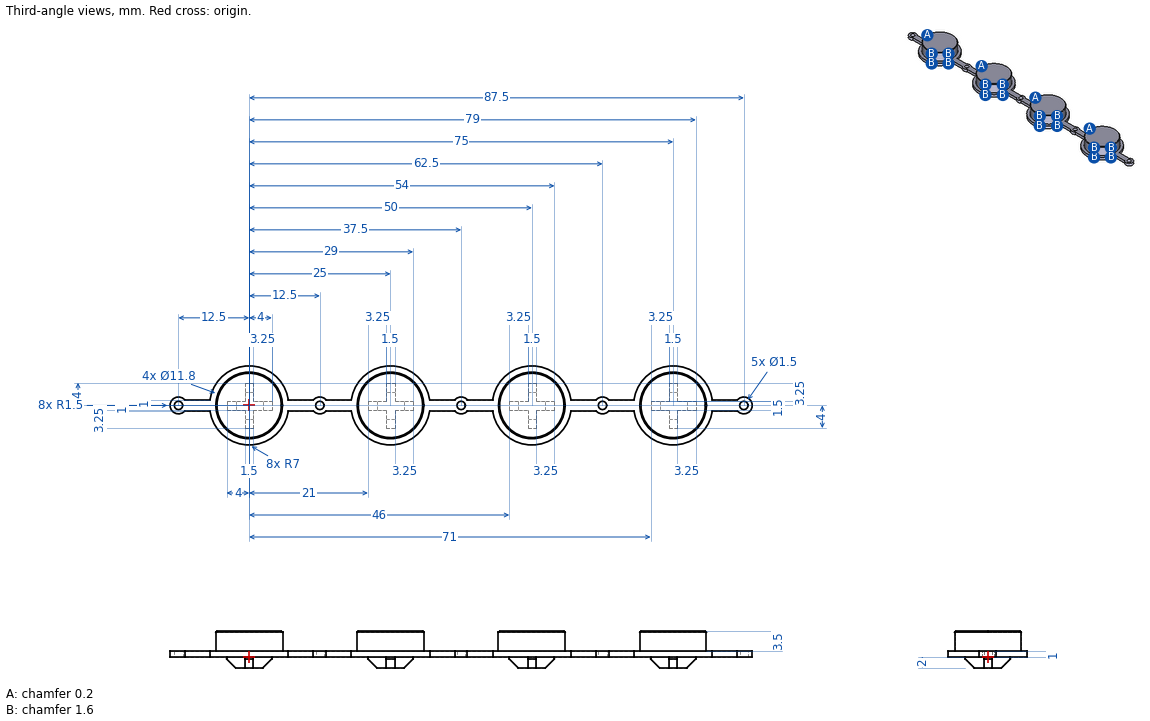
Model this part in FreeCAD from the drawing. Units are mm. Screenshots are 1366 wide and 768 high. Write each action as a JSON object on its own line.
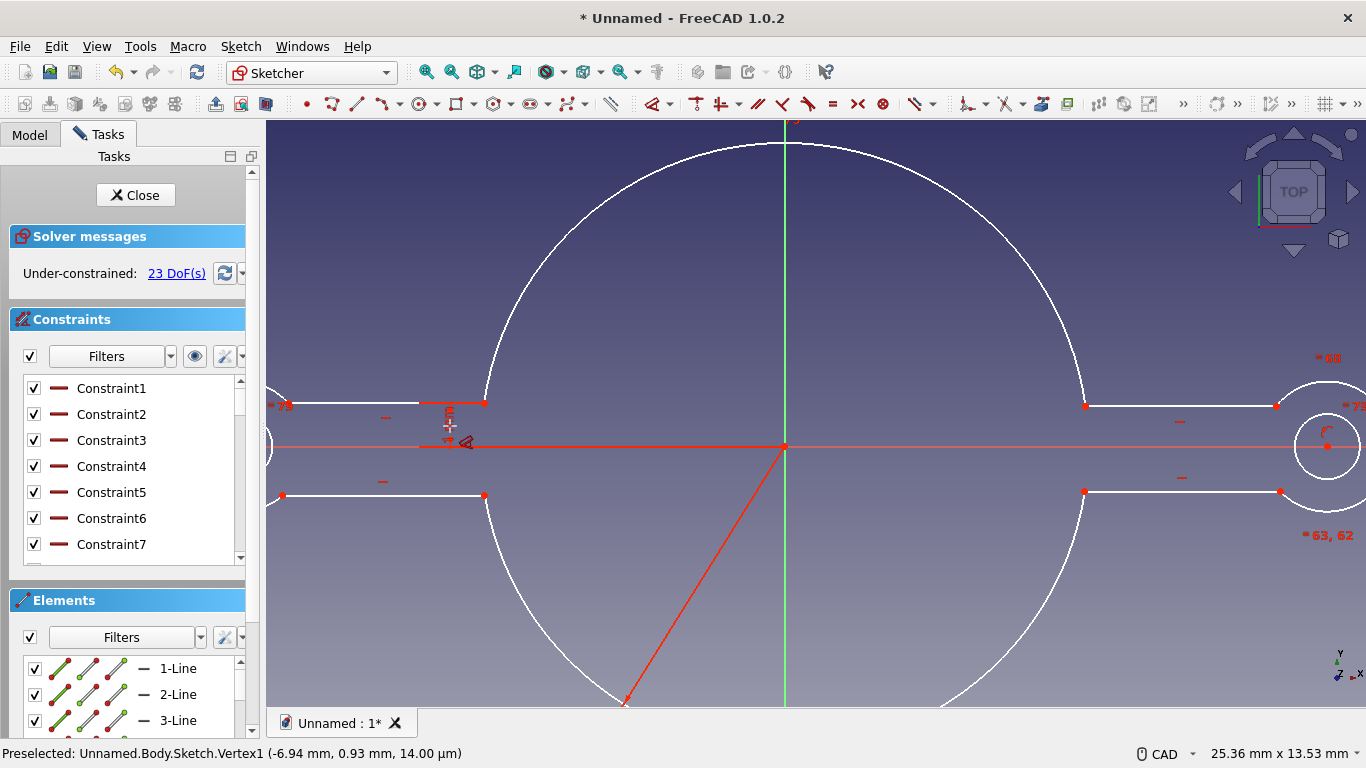
{"action": "scroll", "coordinate": [487, 408], "scroll_direction": "down", "scroll_amount": 10}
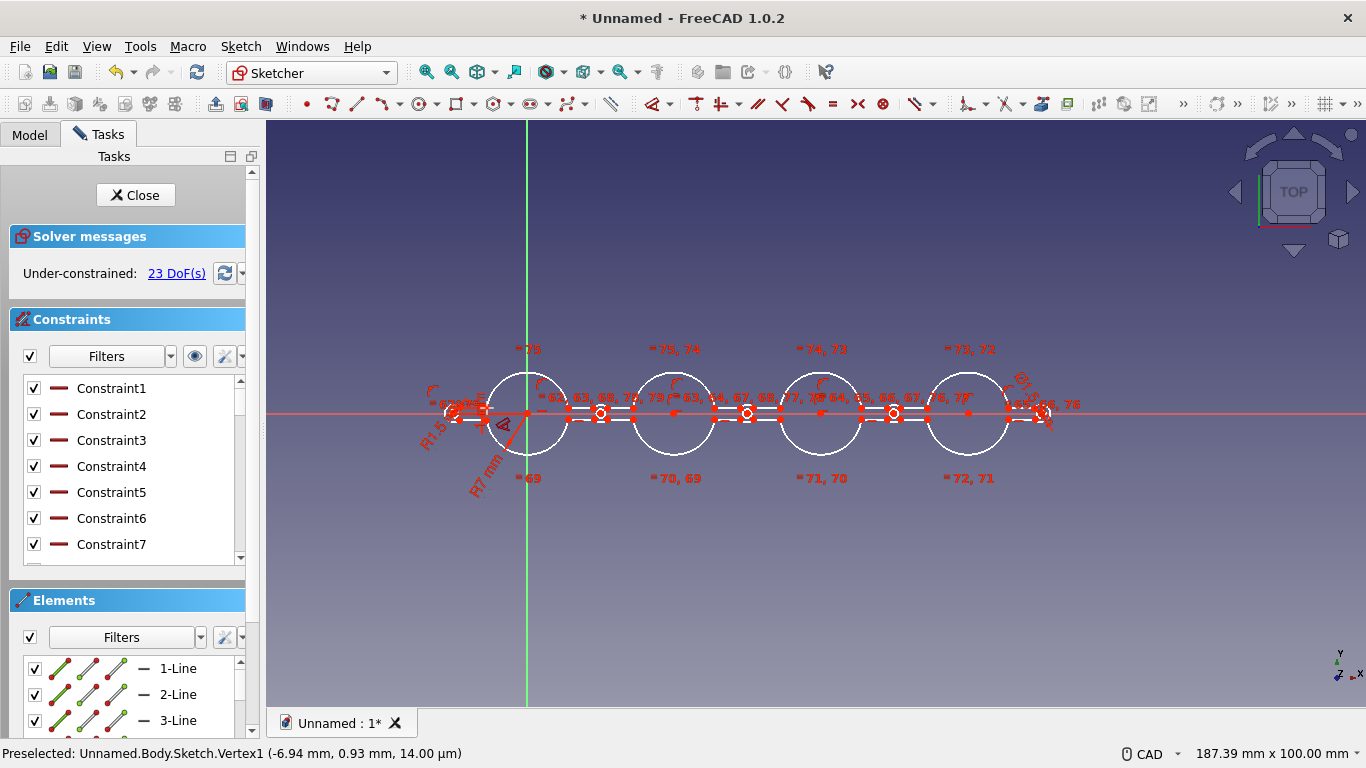
{"action": "scroll", "coordinate": [459, 420], "scroll_direction": "up", "scroll_amount": 10}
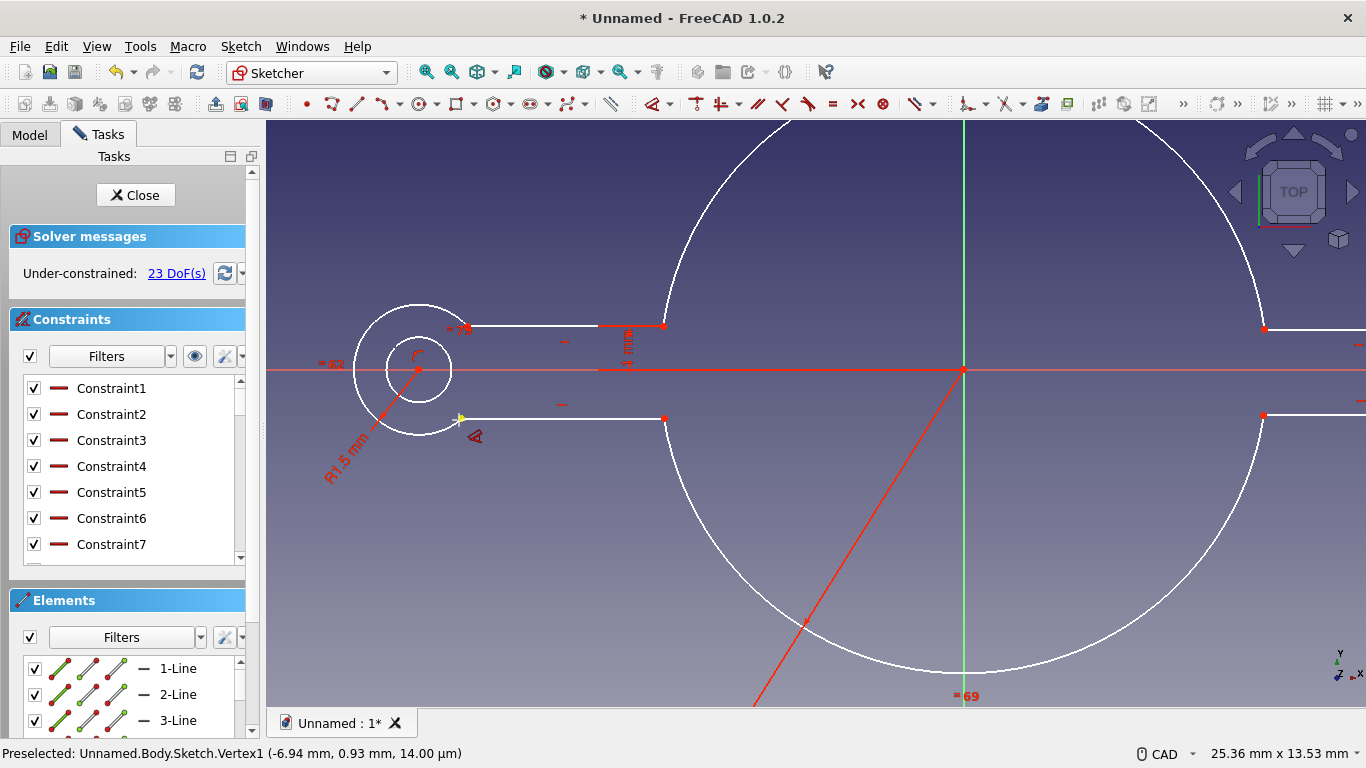
{"action": "left_click", "coordinate": [461, 419]}
{"action": "left_click", "coordinate": [427, 383]}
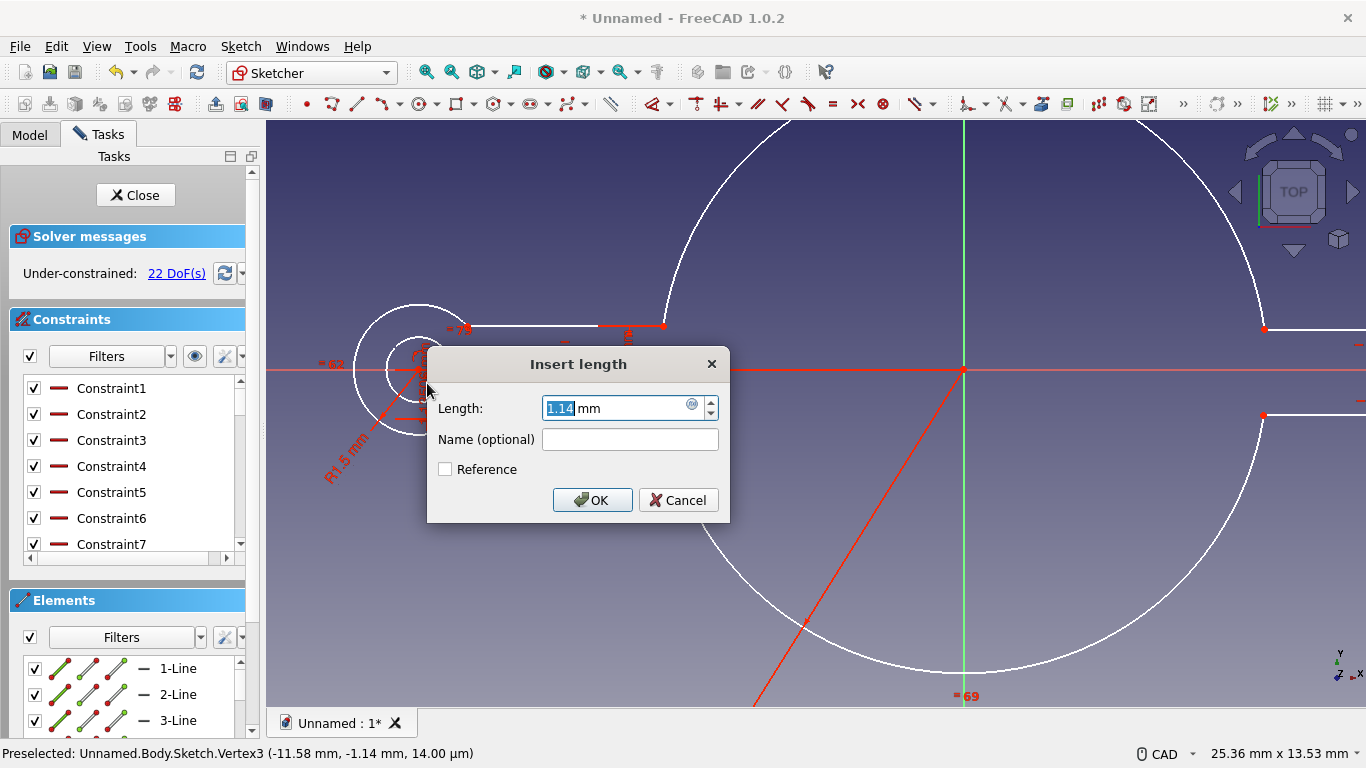
{"action": "type", "text": "1"}
{"action": "key", "text": "Return"}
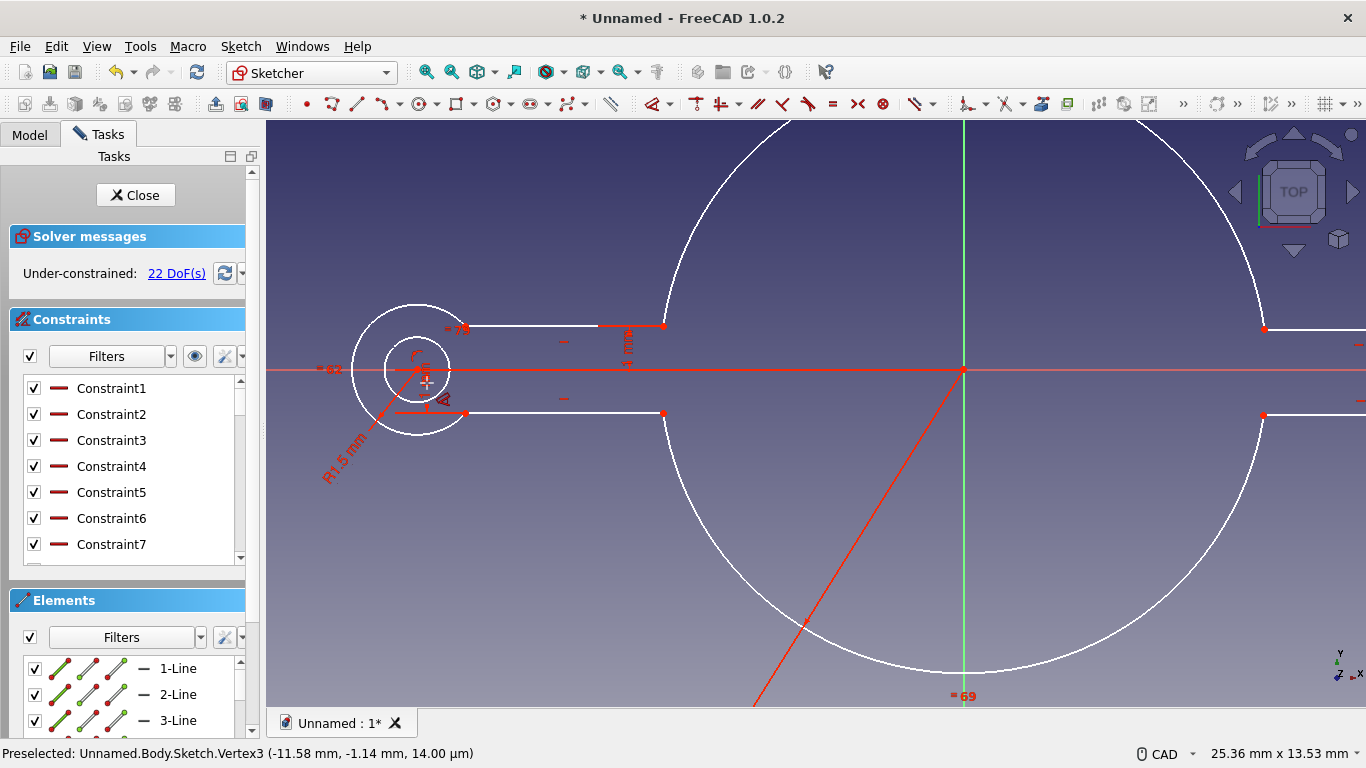
{"action": "scroll", "coordinate": [459, 420], "scroll_direction": "down", "scroll_amount": 10}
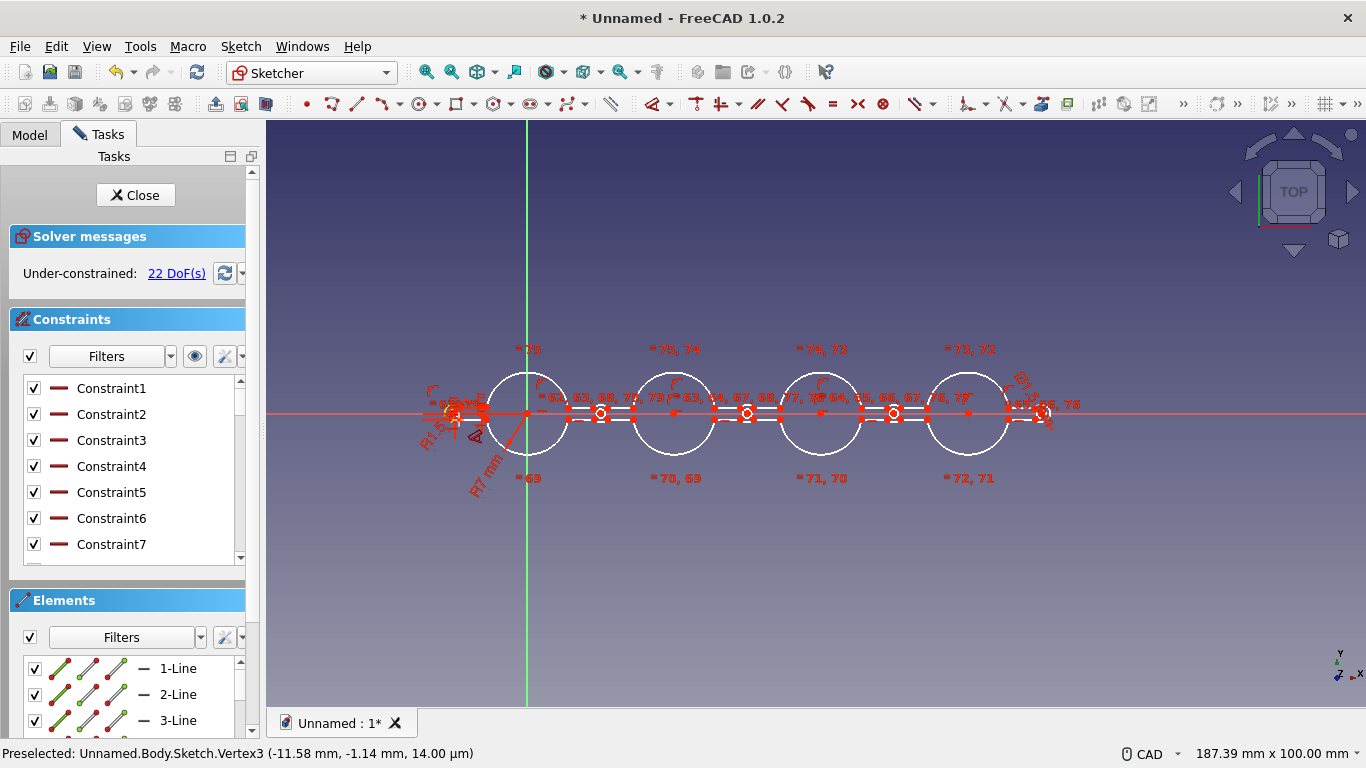
{"action": "scroll", "coordinate": [568, 420], "scroll_direction": "up", "scroll_amount": 10}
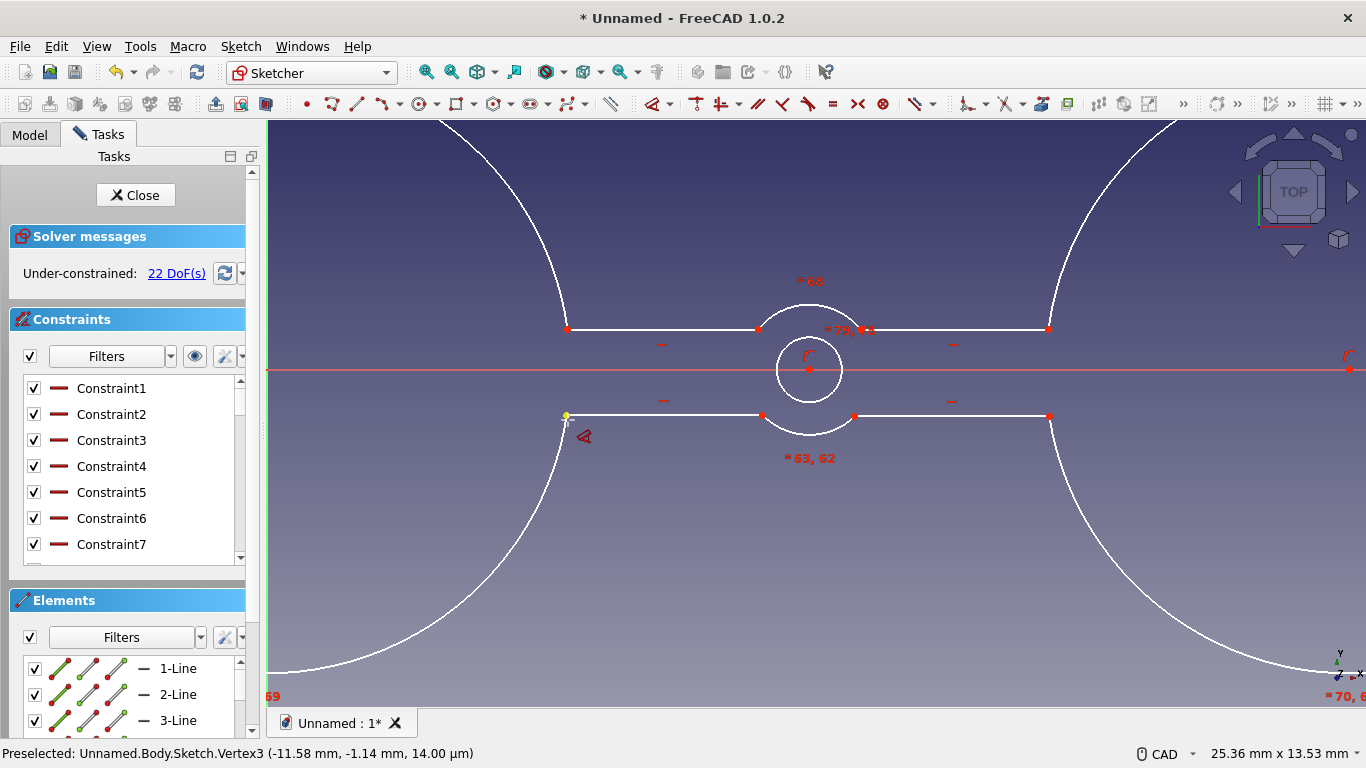
{"action": "left_click", "coordinate": [567, 415]}
{"action": "left_click", "coordinate": [601, 392]}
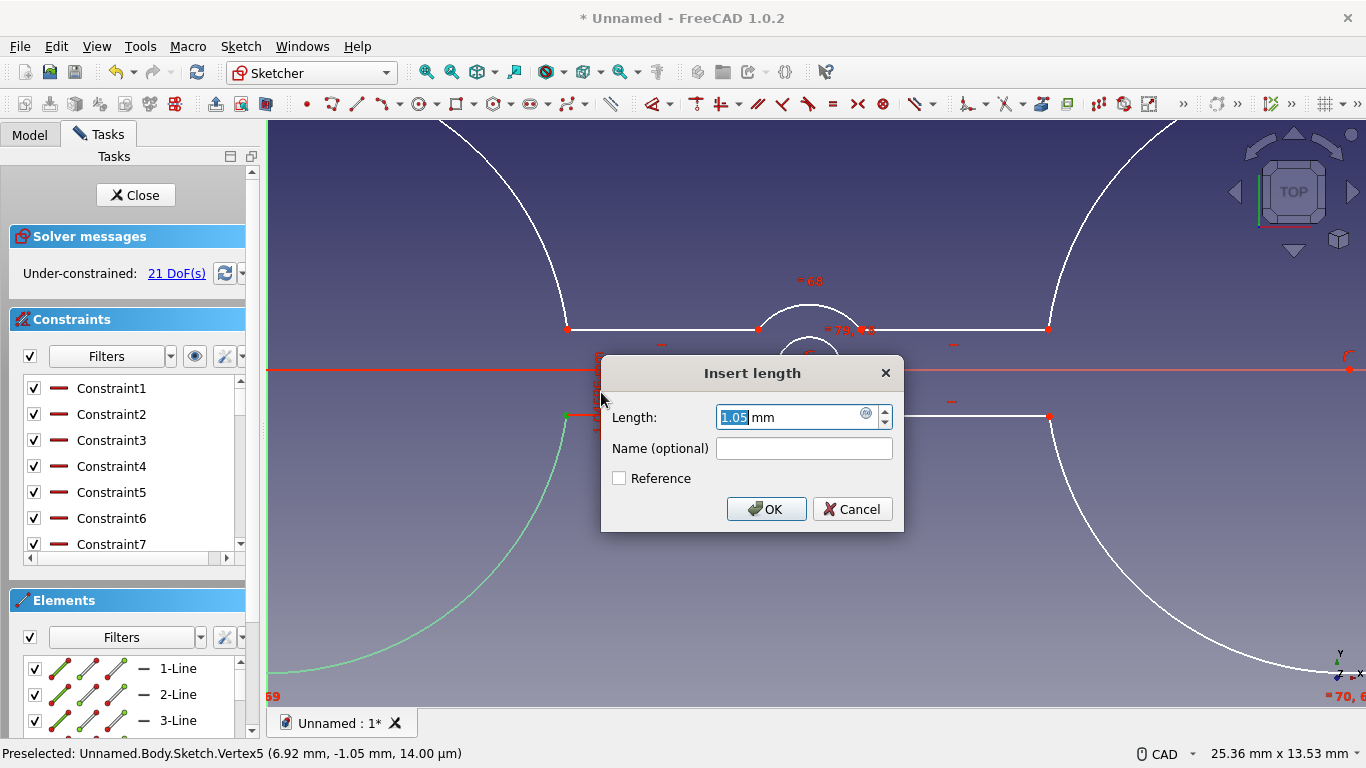
{"action": "type", "text": "1"}
{"action": "key", "text": "Return"}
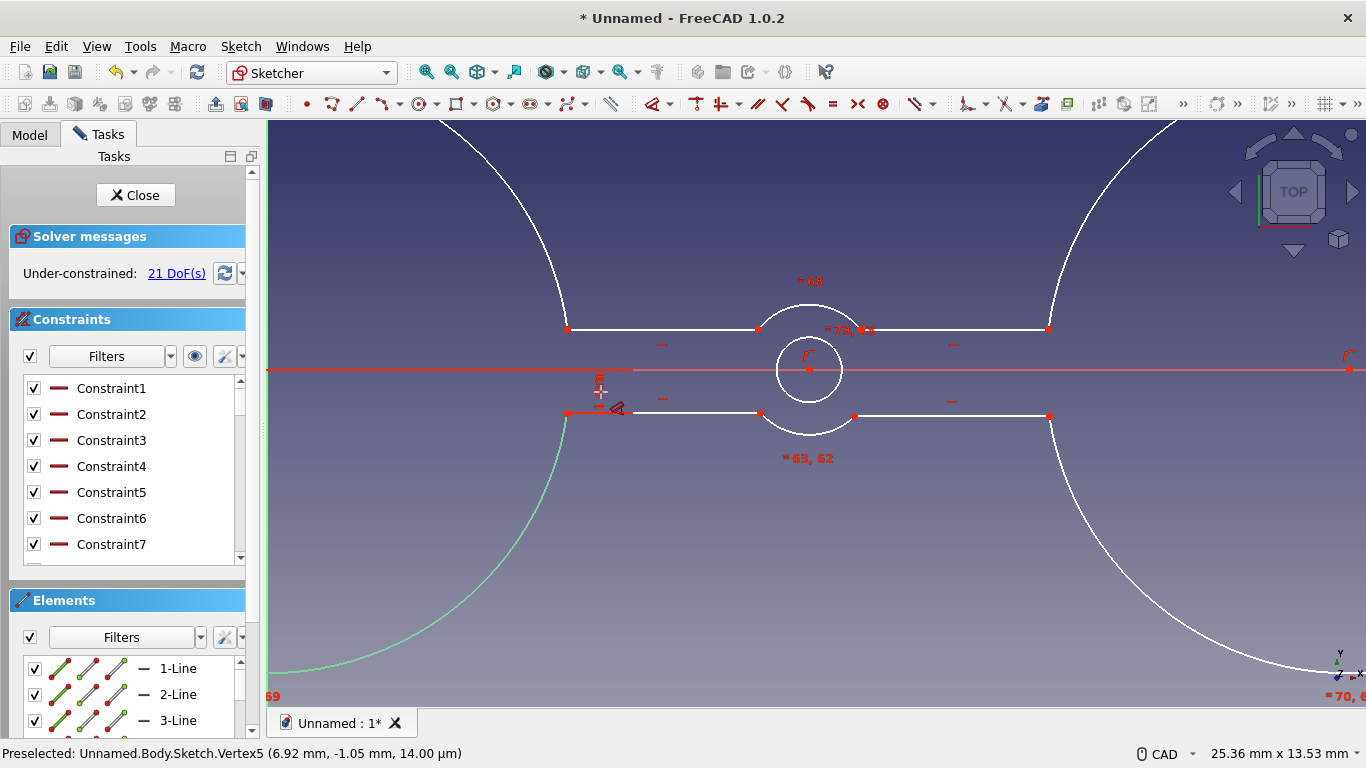
{"action": "left_click", "coordinate": [855, 416]}
{"action": "left_click", "coordinate": [889, 393]}